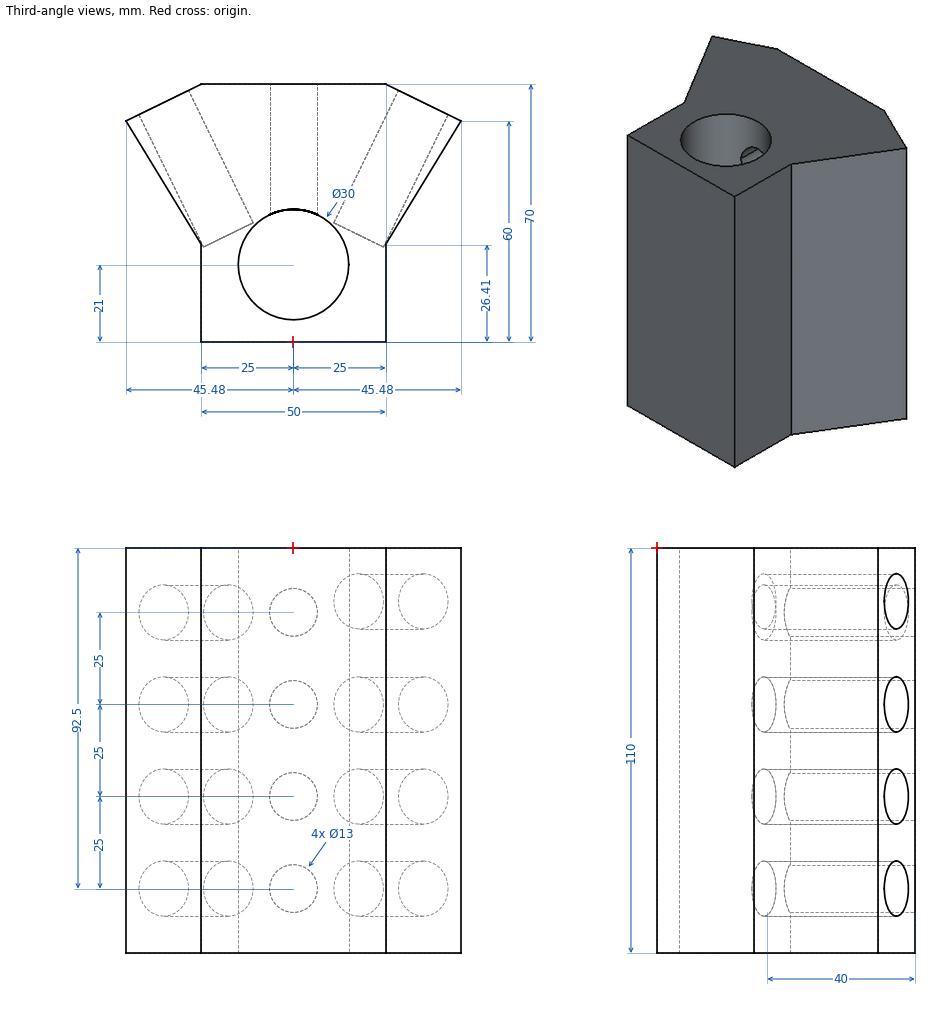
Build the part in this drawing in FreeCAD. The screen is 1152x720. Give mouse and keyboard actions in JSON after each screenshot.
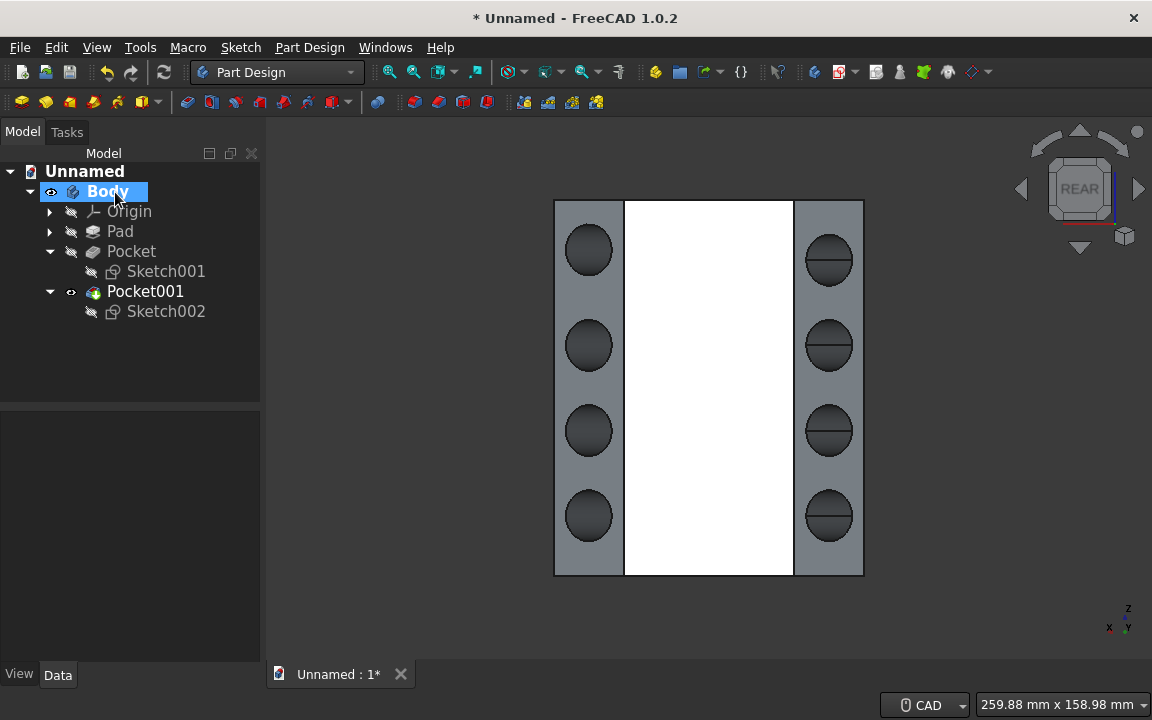
{"action": "left_click", "coordinate": [709, 333]}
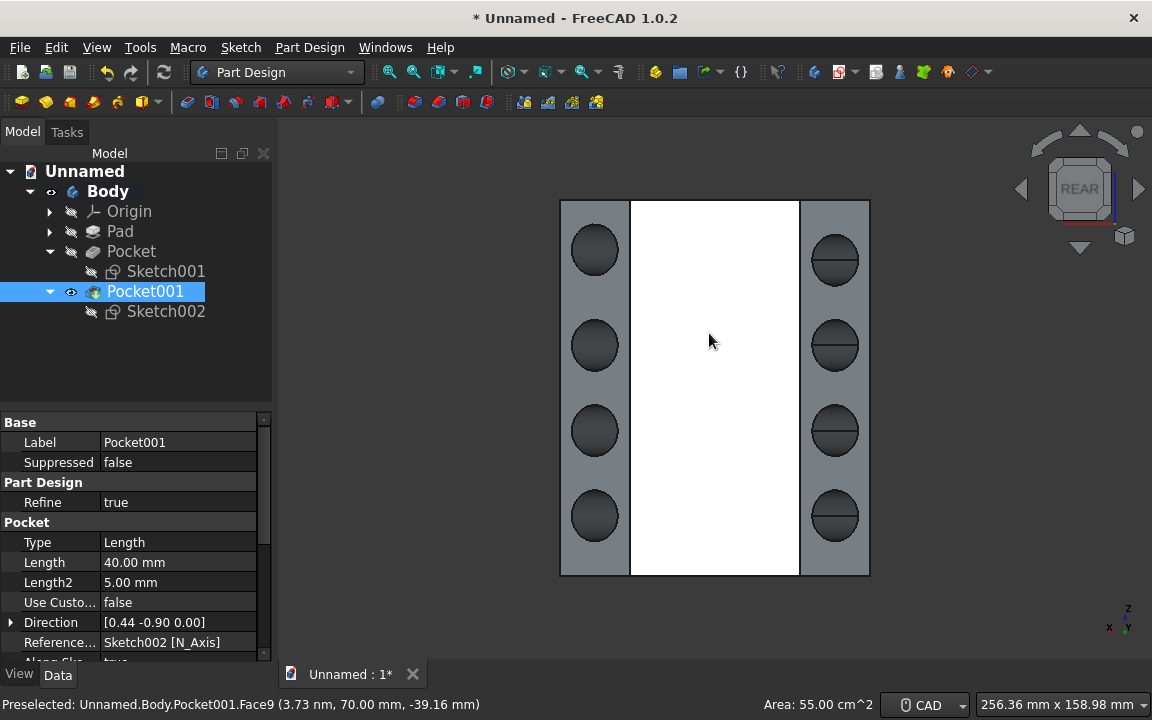
{"action": "left_click", "coordinate": [840, 72]}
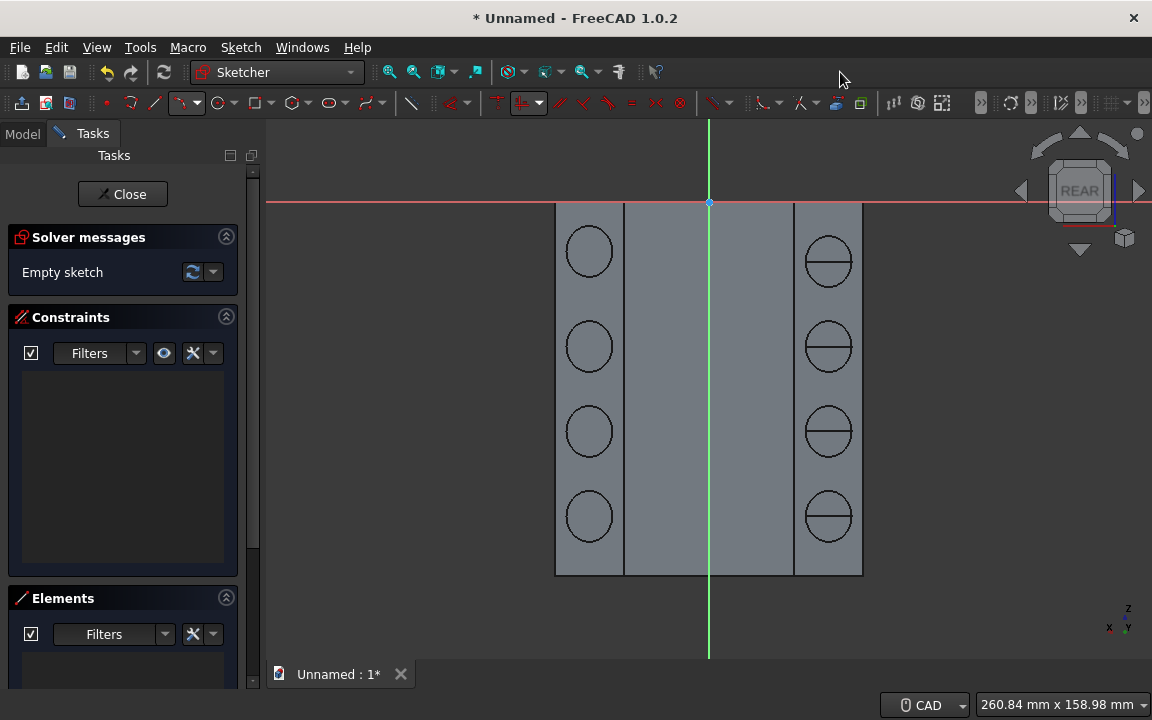
{"action": "left_click", "coordinate": [218, 104]}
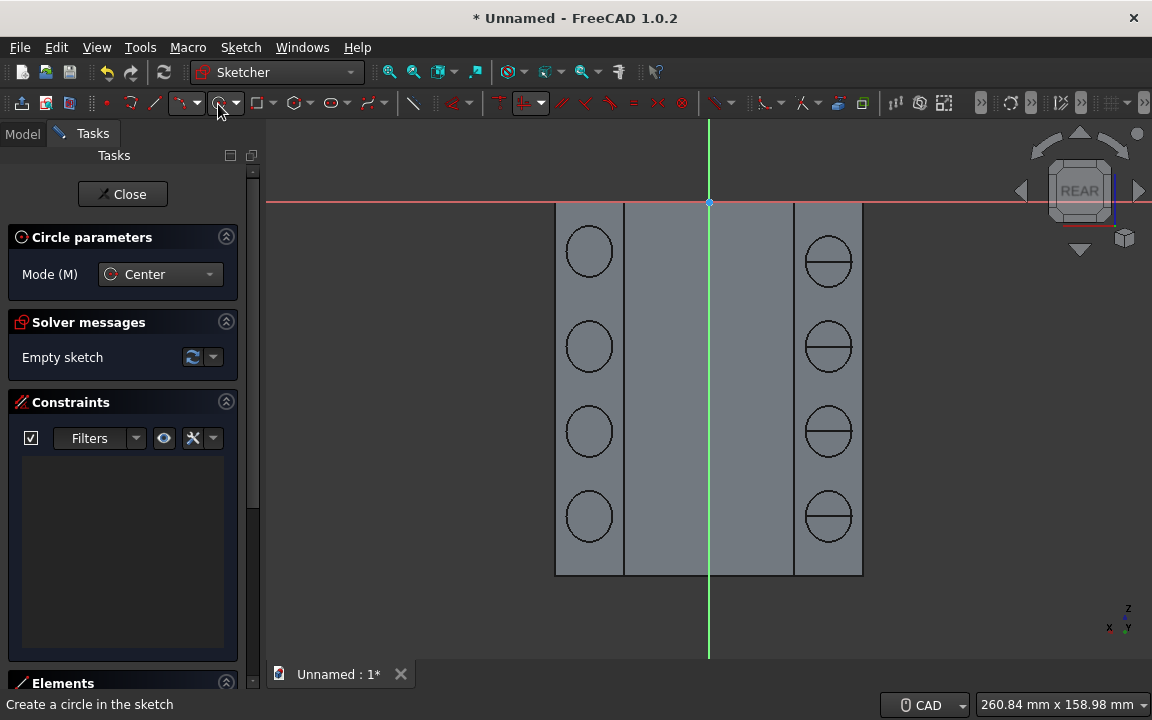
{"action": "left_click", "coordinate": [709, 516]}
{"action": "left_click", "coordinate": [725, 501]}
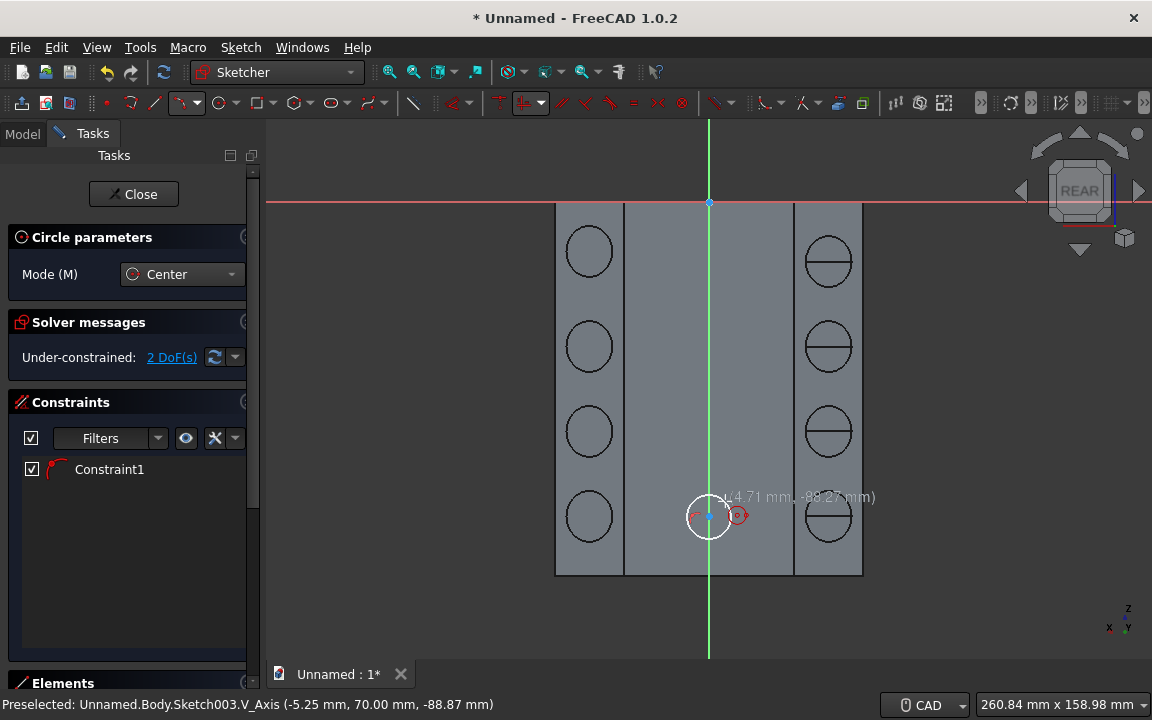
{"action": "left_click", "coordinate": [709, 431]}
{"action": "left_click", "coordinate": [725, 416]}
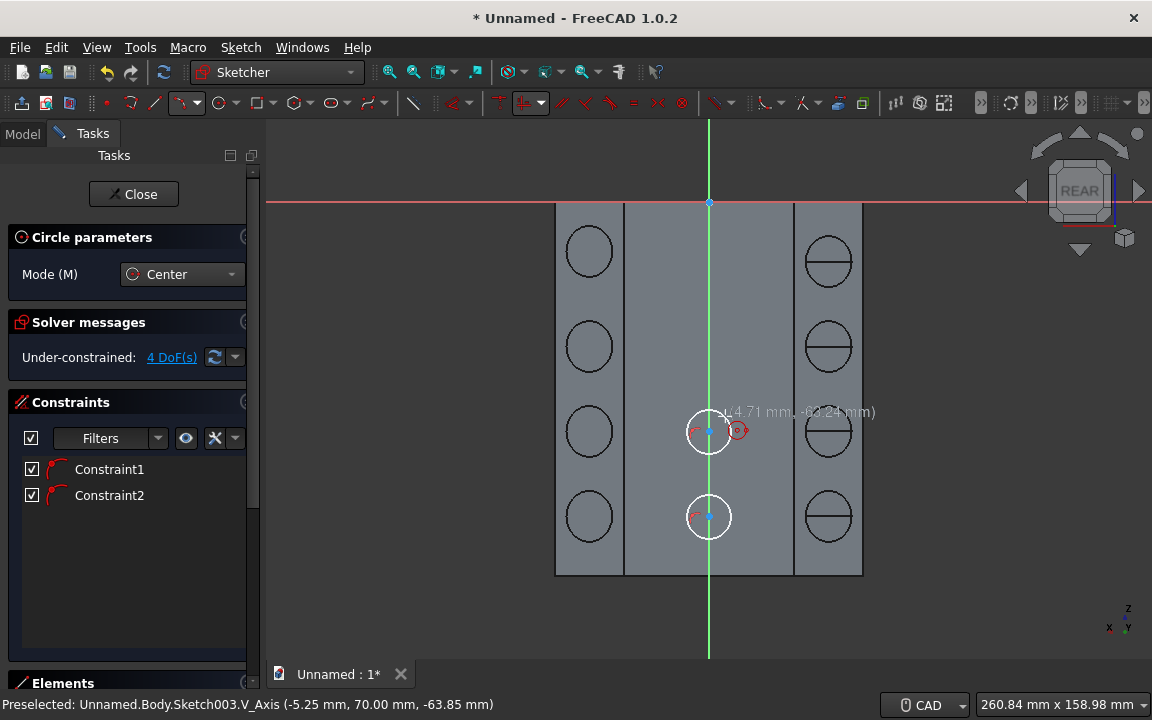
{"action": "left_click", "coordinate": [709, 347]}
{"action": "left_click", "coordinate": [725, 331]}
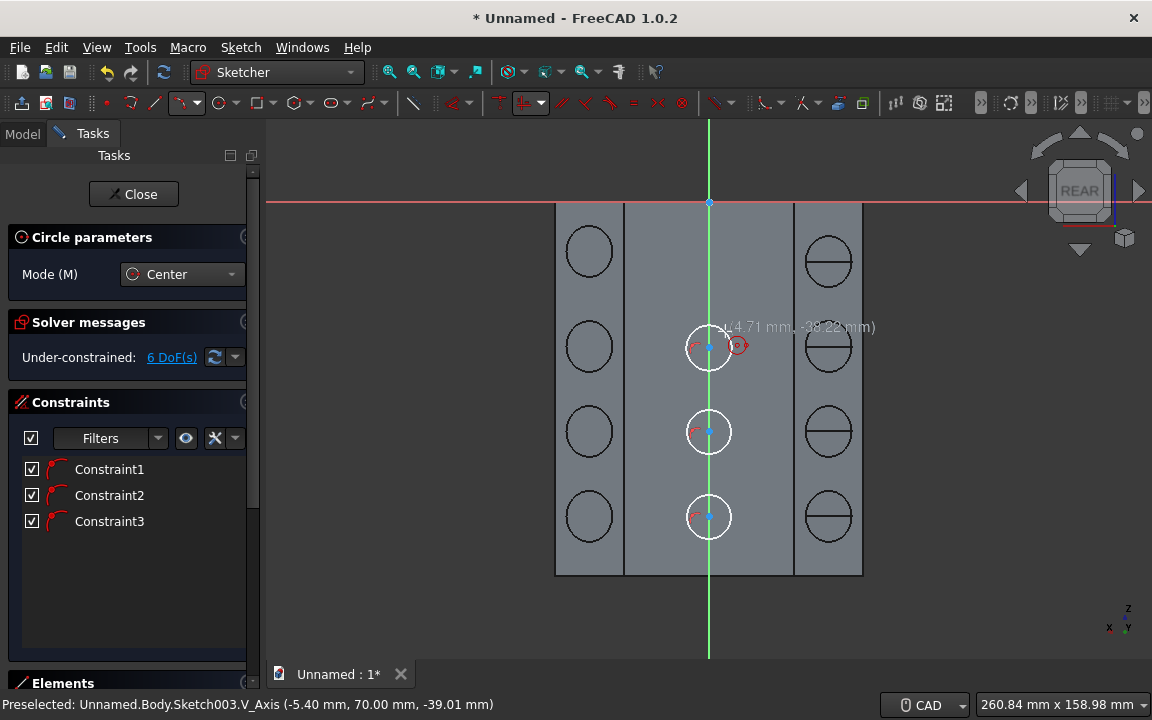
{"action": "left_click", "coordinate": [709, 262]}
{"action": "left_click", "coordinate": [725, 246]}
{"action": "key", "text": "Escape"}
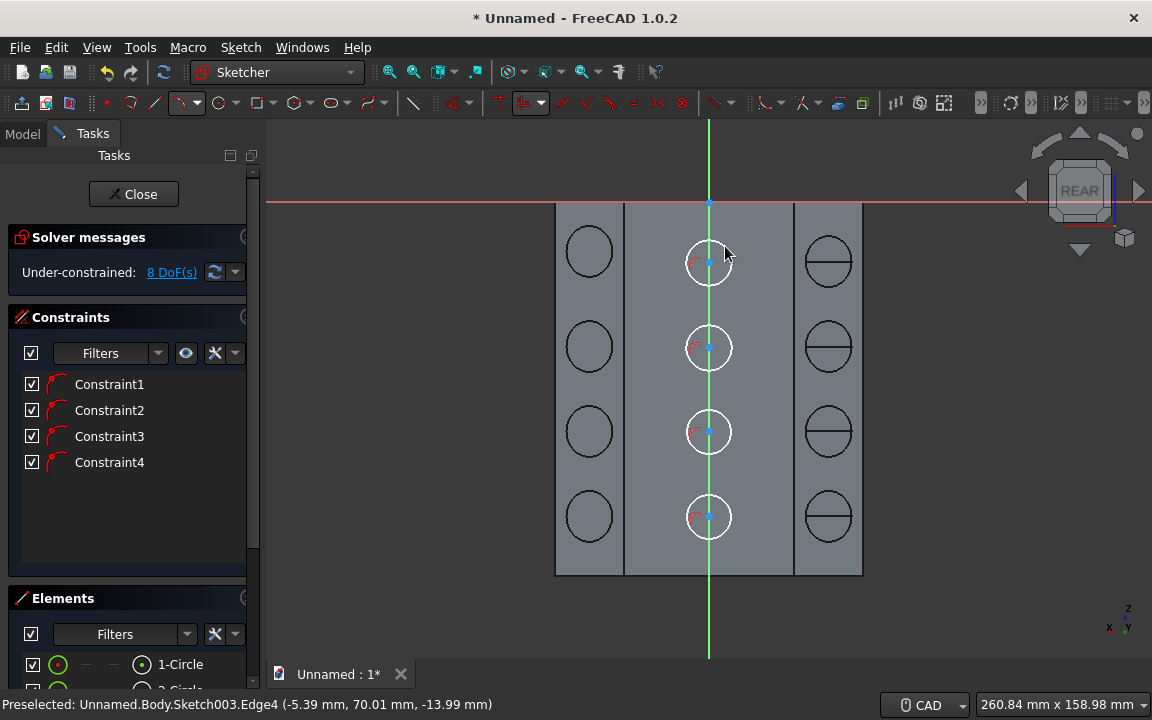
{"action": "left_click", "coordinate": [724, 501]}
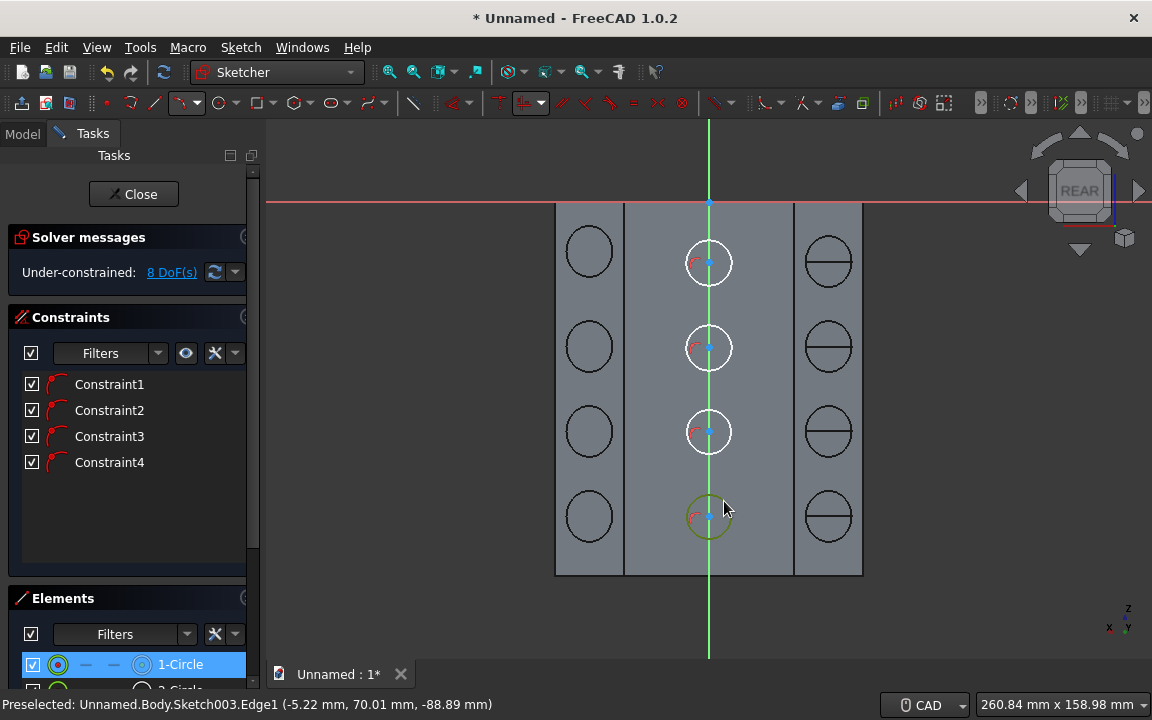
{"action": "left_click", "coordinate": [724, 416]}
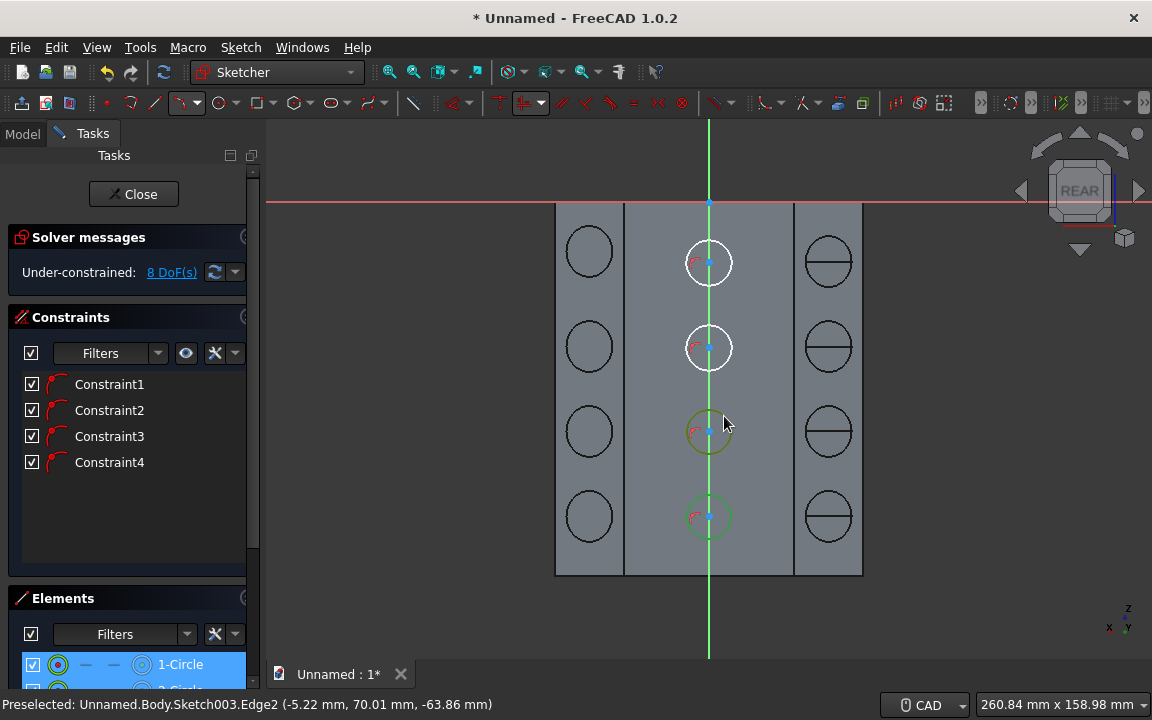
{"action": "left_click", "coordinate": [725, 332]}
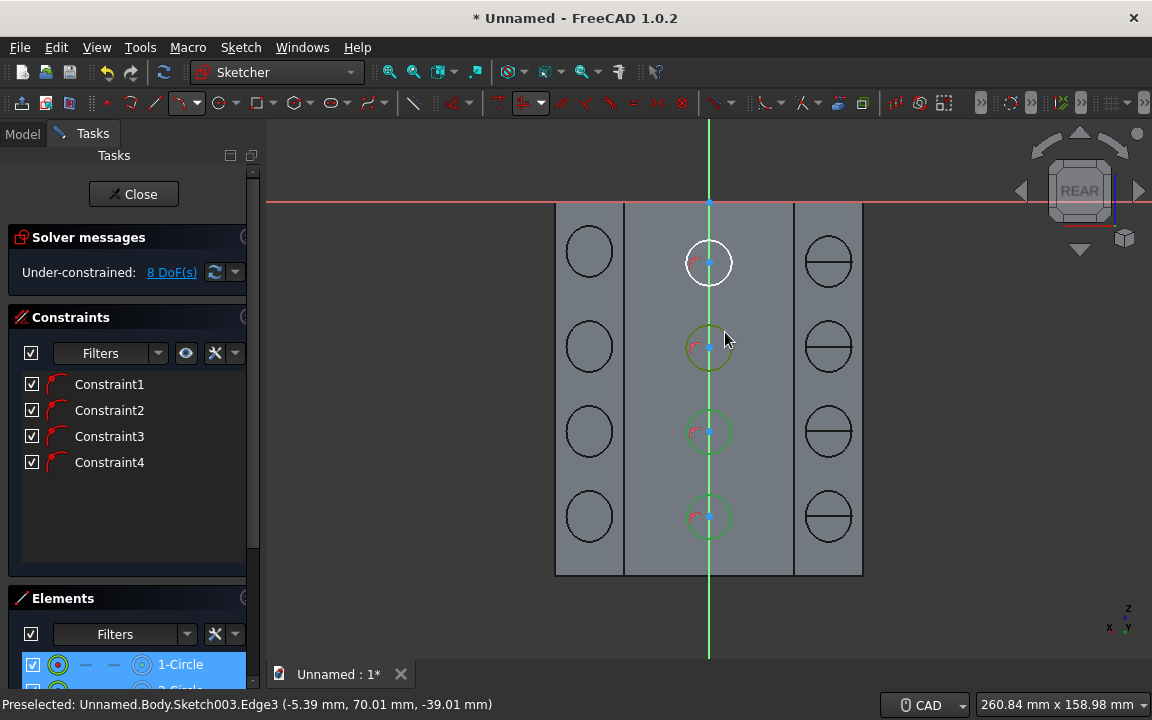
{"action": "left_click", "coordinate": [725, 247]}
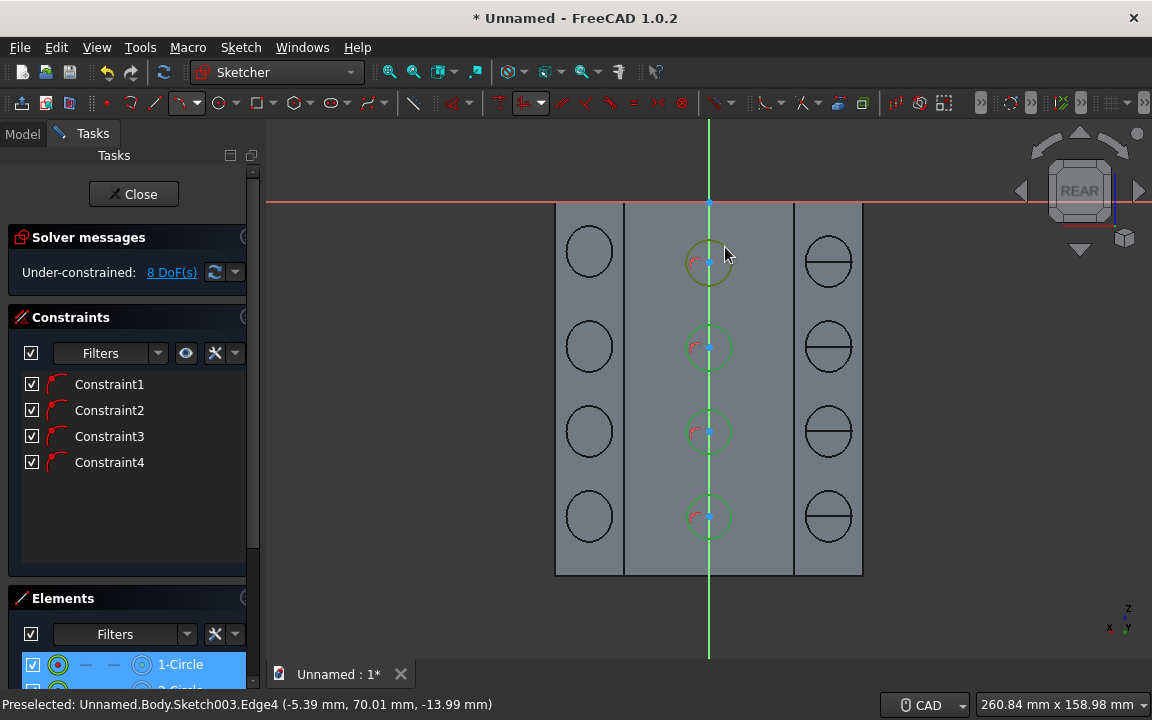
{"action": "left_click", "coordinate": [634, 104]}